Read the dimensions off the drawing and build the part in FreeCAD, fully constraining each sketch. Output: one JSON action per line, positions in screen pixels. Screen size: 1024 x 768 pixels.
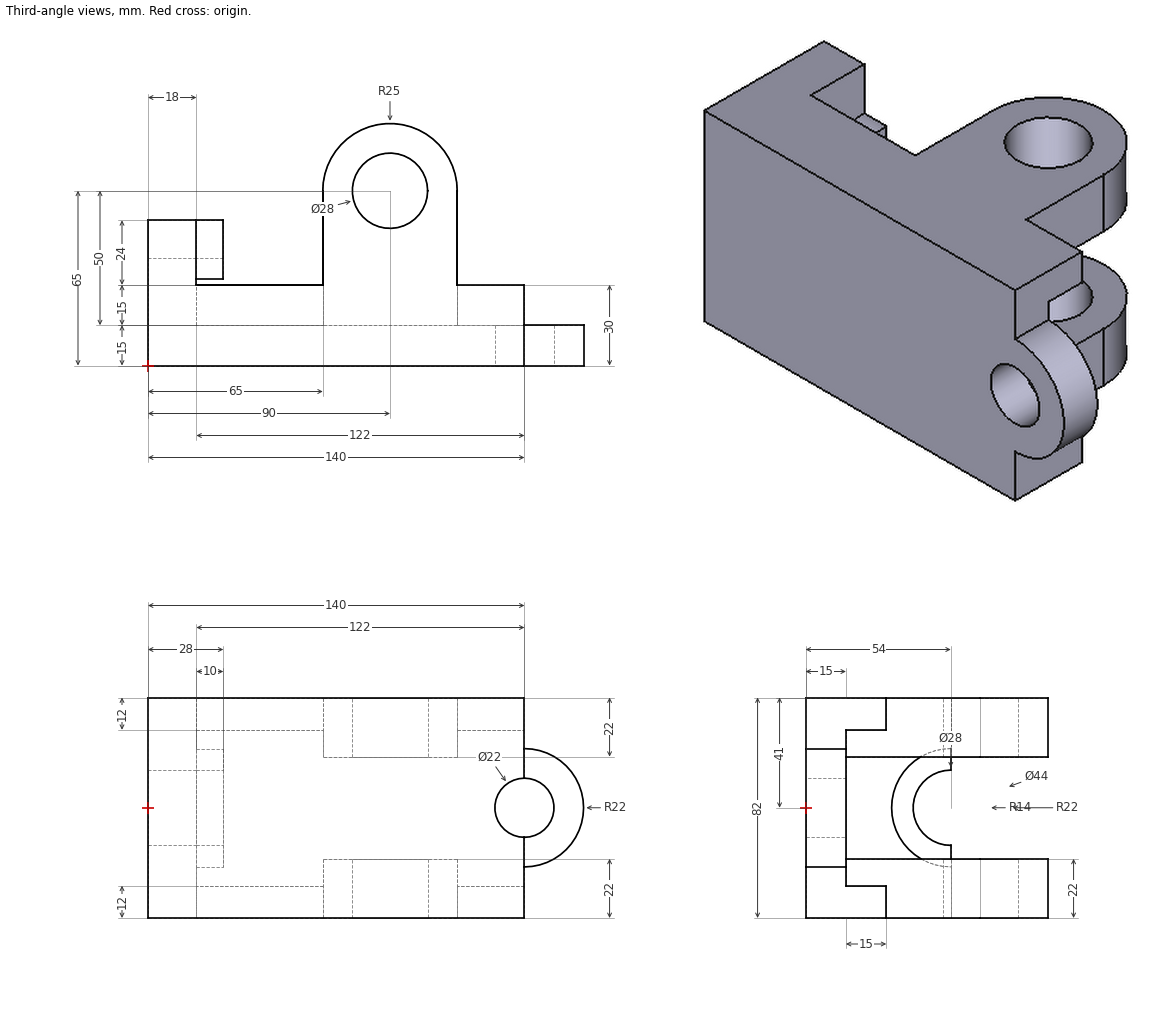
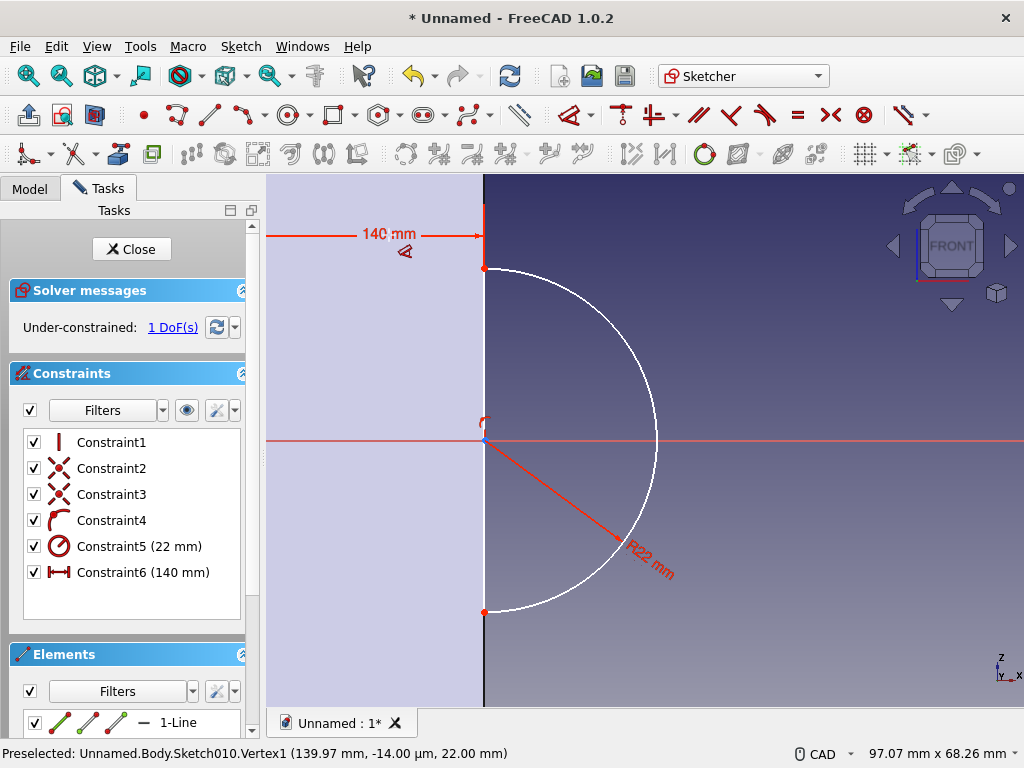
{"action": "left_click", "coordinate": [485, 440]}
{"action": "left_click", "coordinate": [390, 474]}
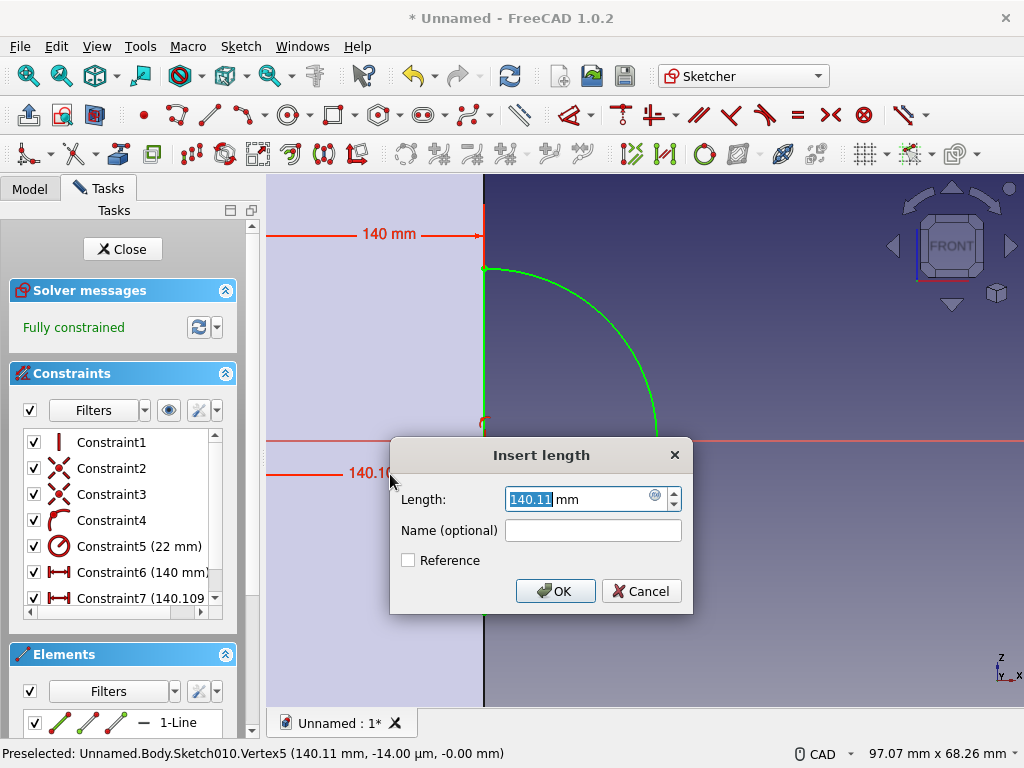
{"action": "type", "text": "140"}
{"action": "key", "text": "Return"}
{"action": "key", "text": "Escape"}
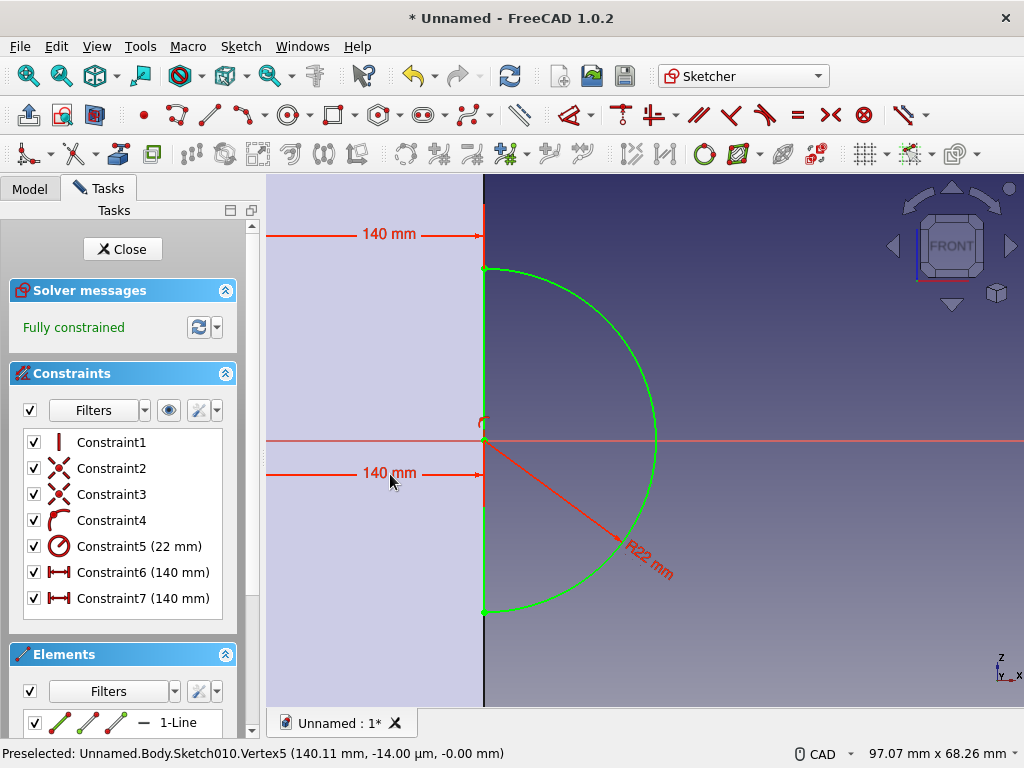
{"action": "left_click", "coordinate": [123, 249]}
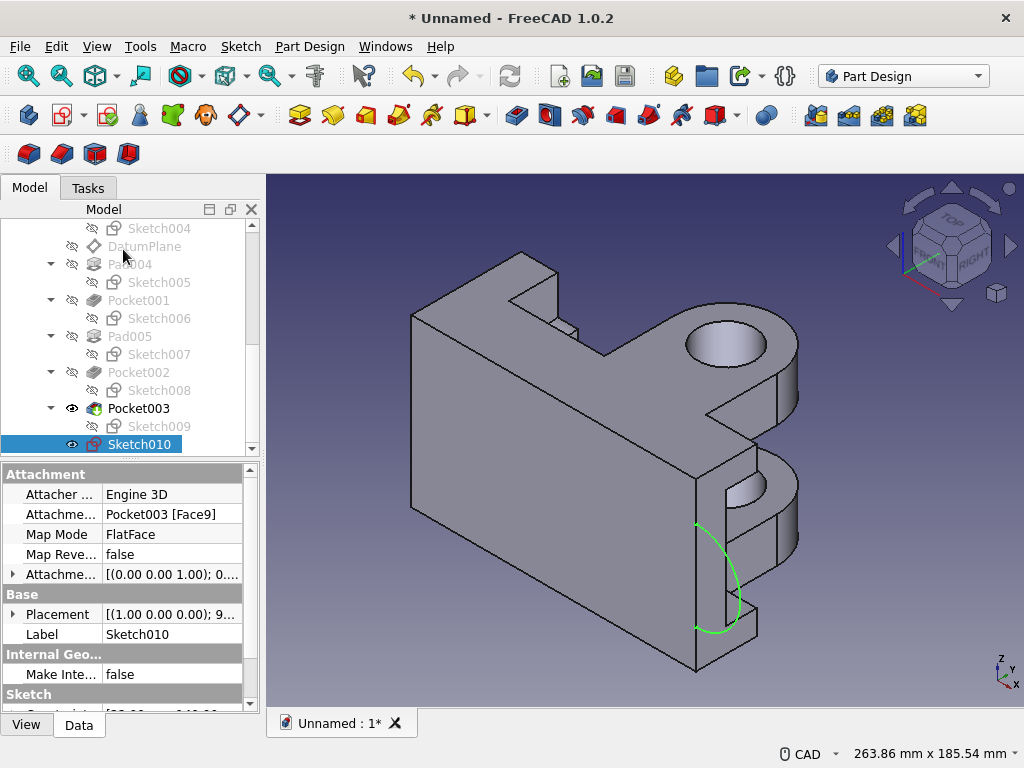
{"action": "left_click", "coordinate": [300, 116]}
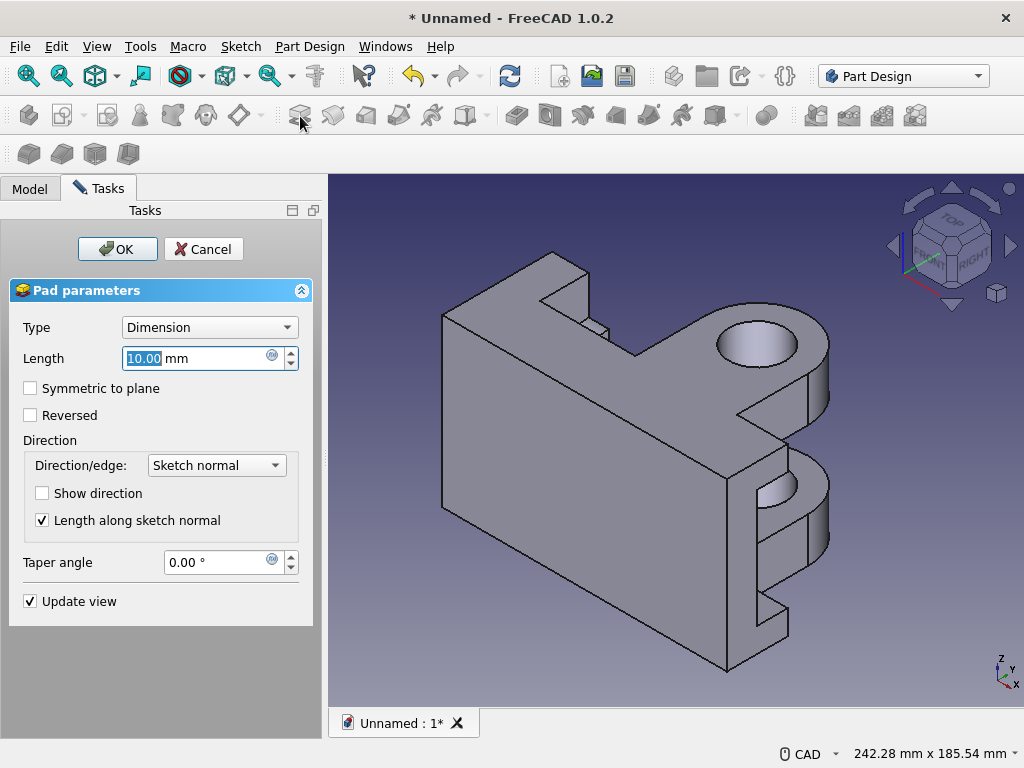
{"action": "type", "text": "15"}
{"action": "key", "text": "Tab"}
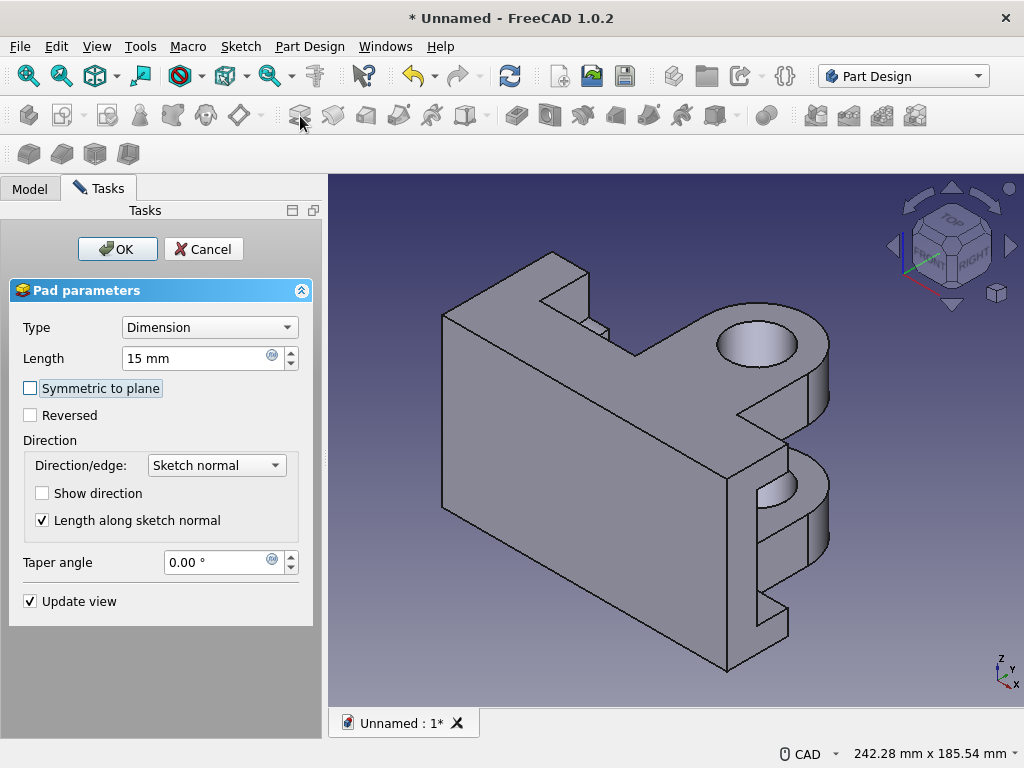
{"action": "left_click", "coordinate": [31, 415]}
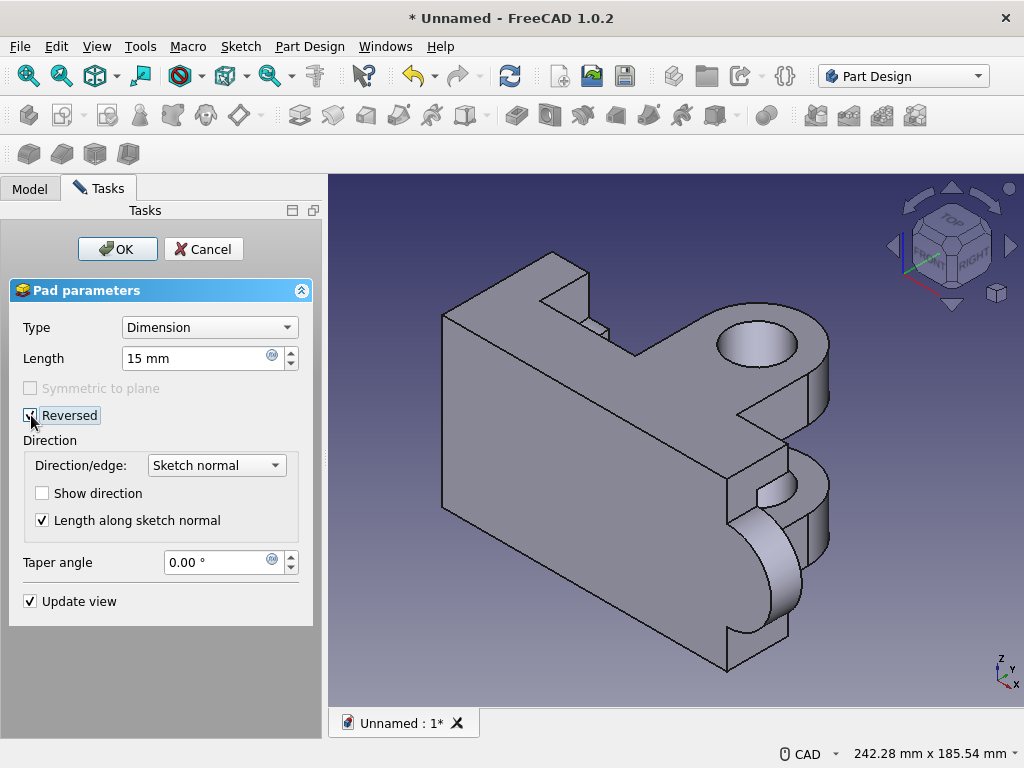
{"action": "left_click", "coordinate": [118, 249]}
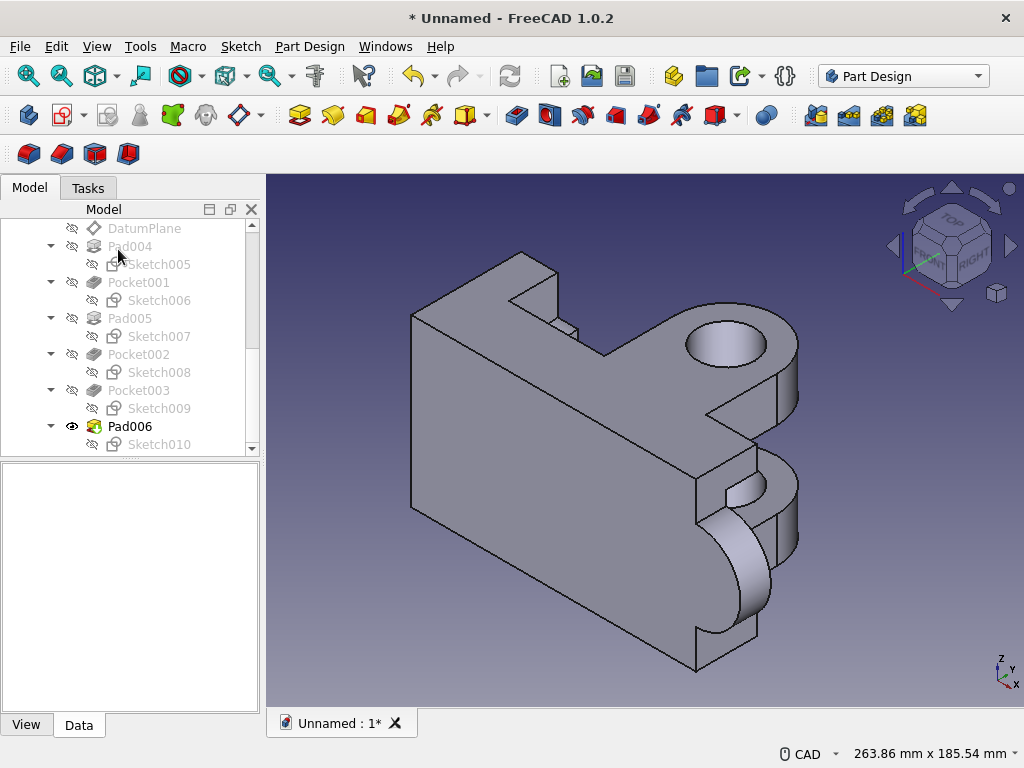
{"action": "left_click", "coordinate": [623, 532]}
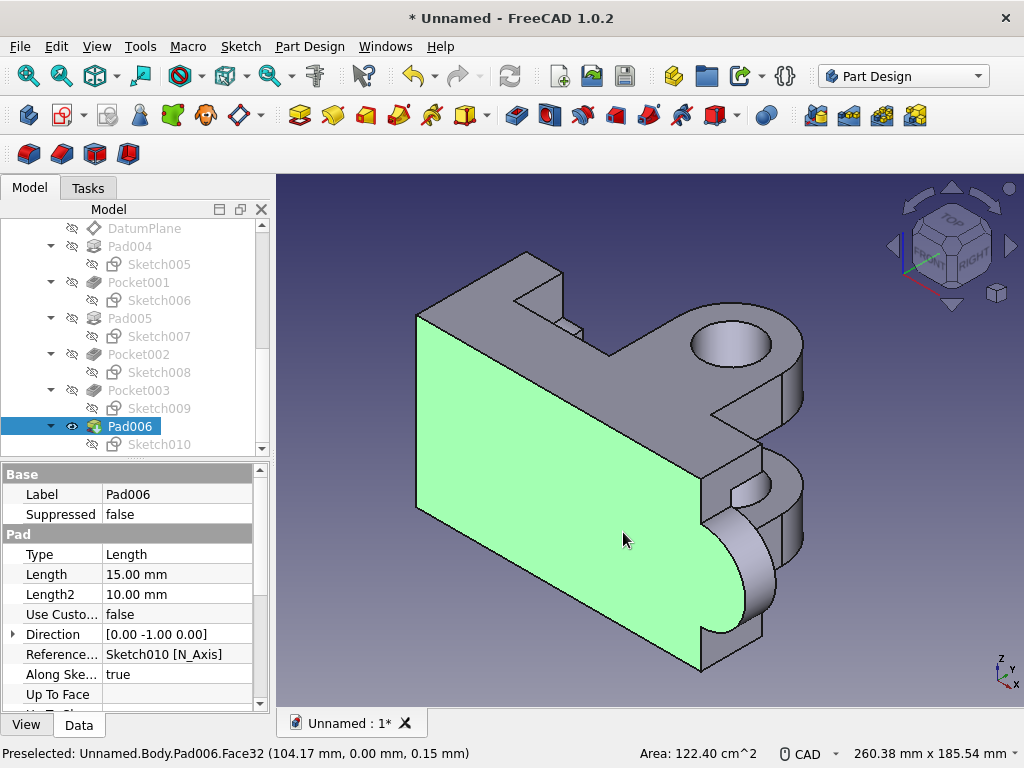
{"action": "left_click", "coordinate": [62, 116]}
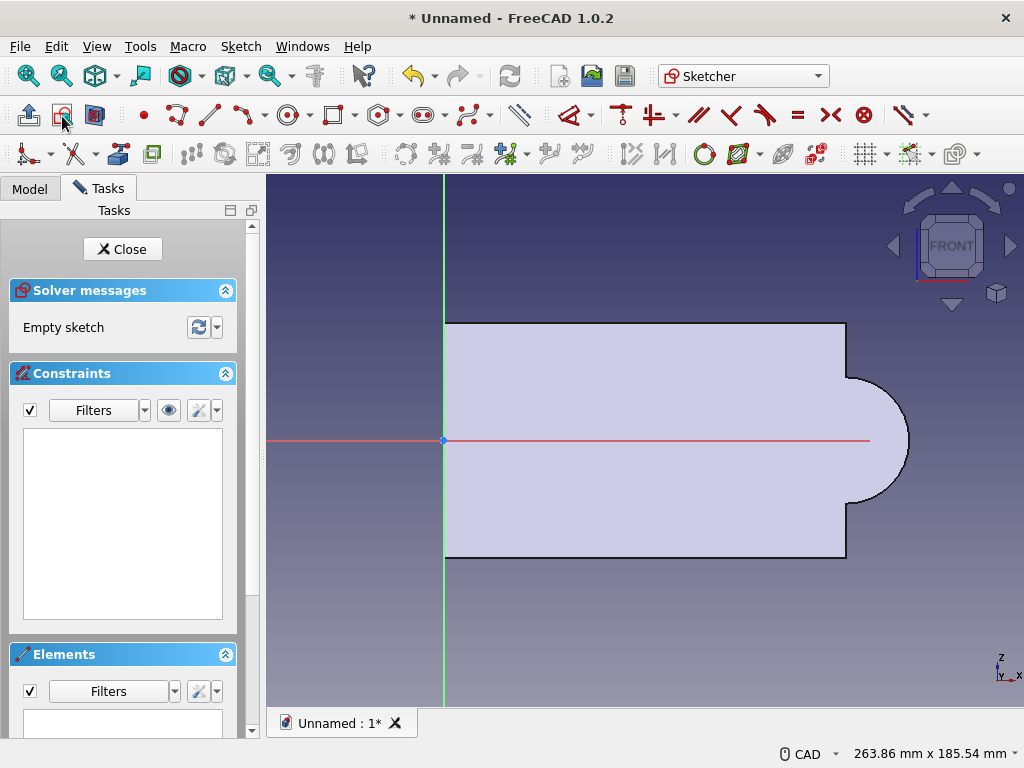
{"action": "scroll", "coordinate": [576, 440], "scroll_direction": "down", "scroll_amount": 5}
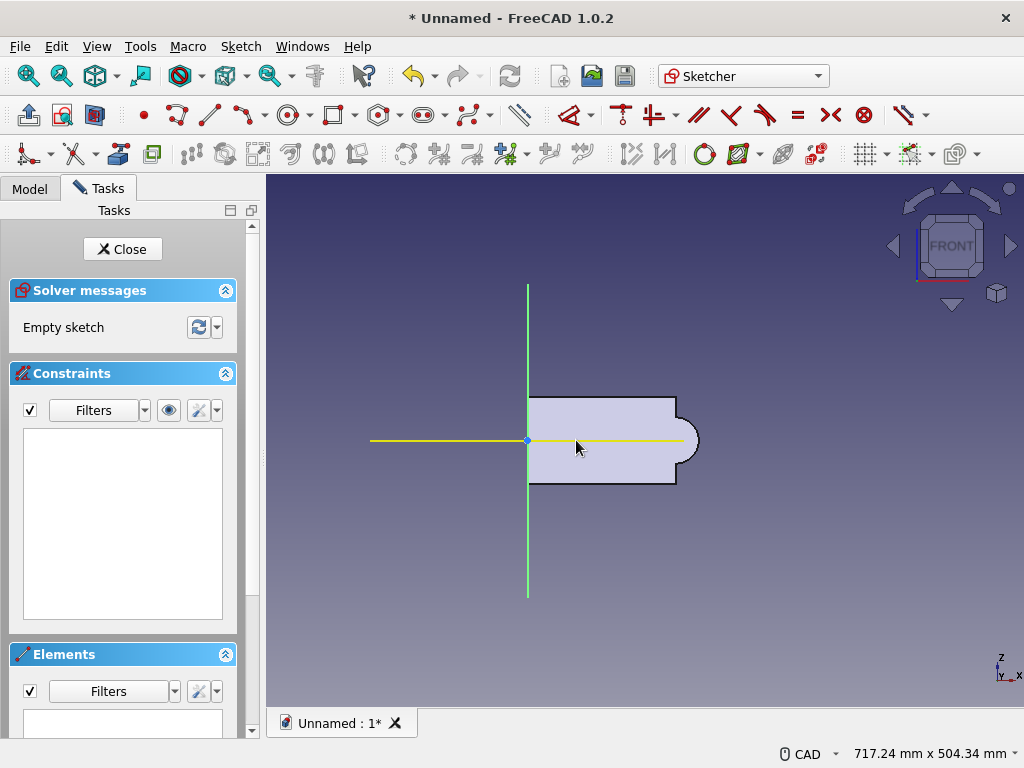
{"action": "scroll", "coordinate": [684, 440], "scroll_direction": "up", "scroll_amount": 13}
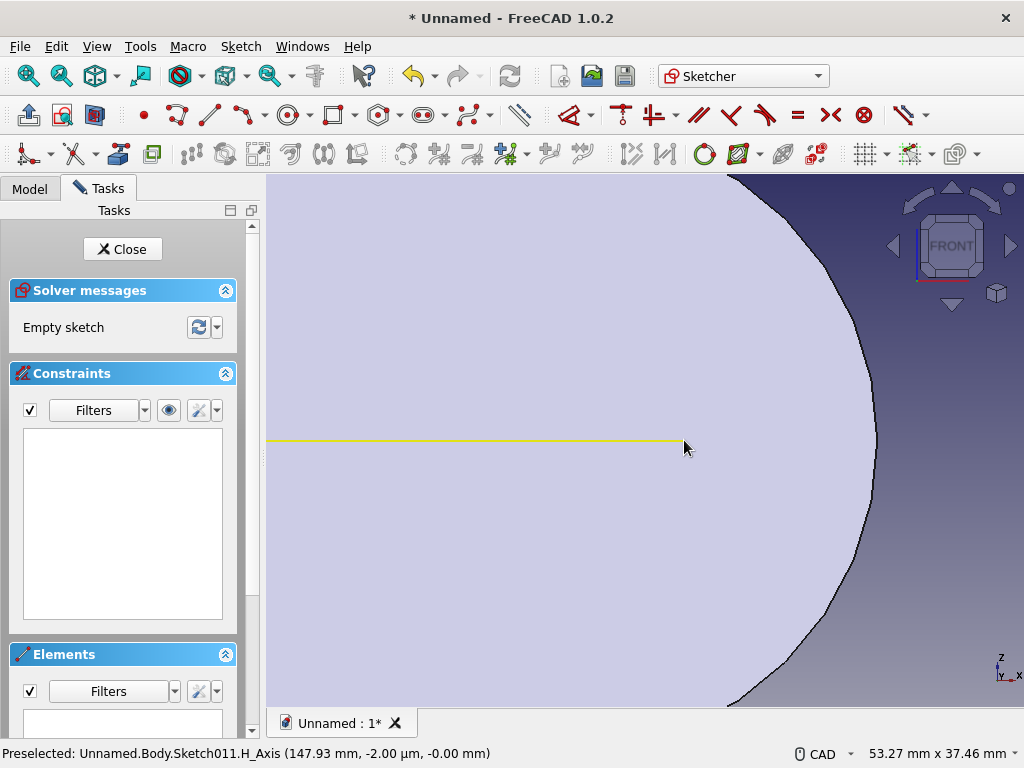
{"action": "left_click", "coordinate": [288, 116]}